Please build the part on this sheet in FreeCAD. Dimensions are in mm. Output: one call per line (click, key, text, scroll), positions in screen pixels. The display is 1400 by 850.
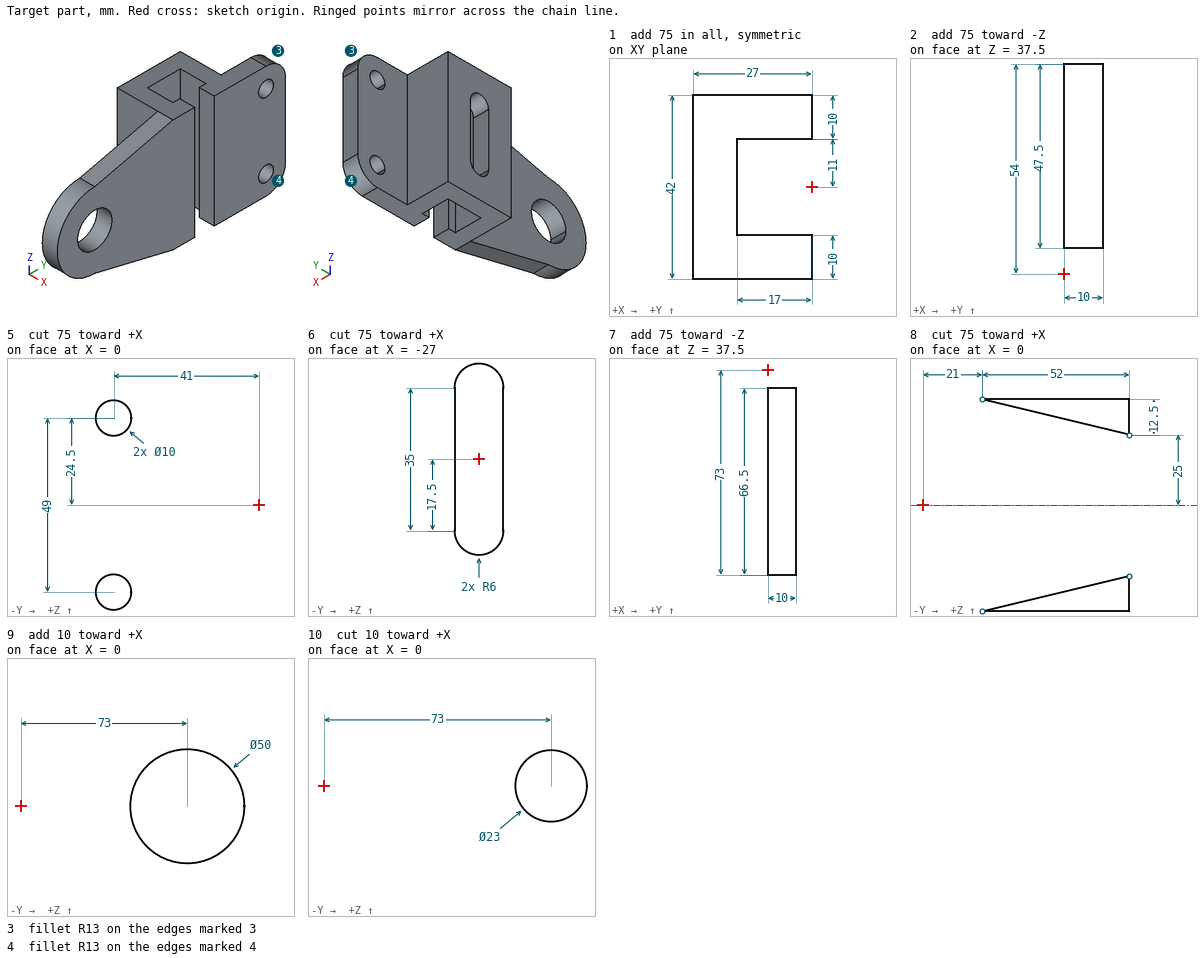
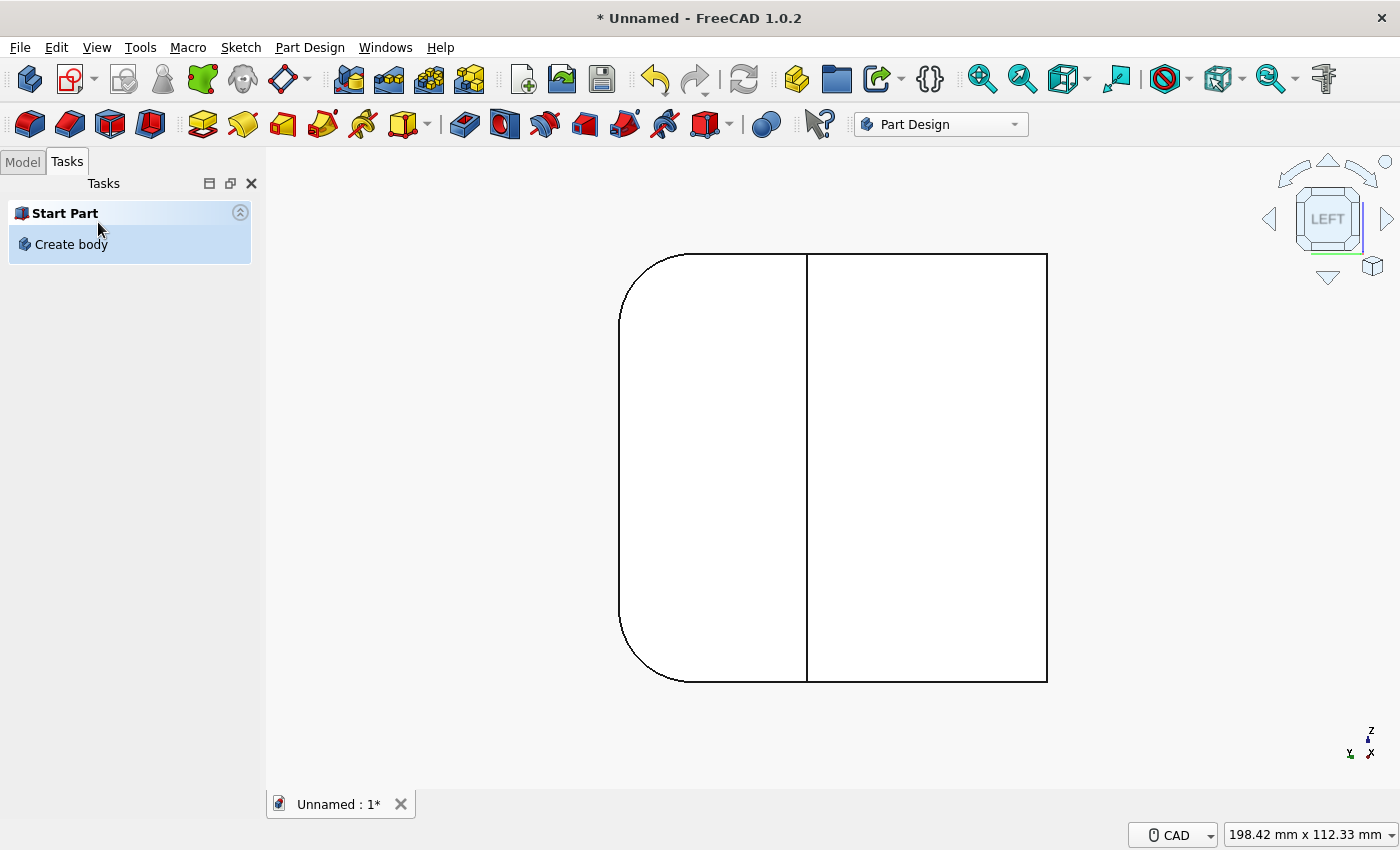
click(713, 406)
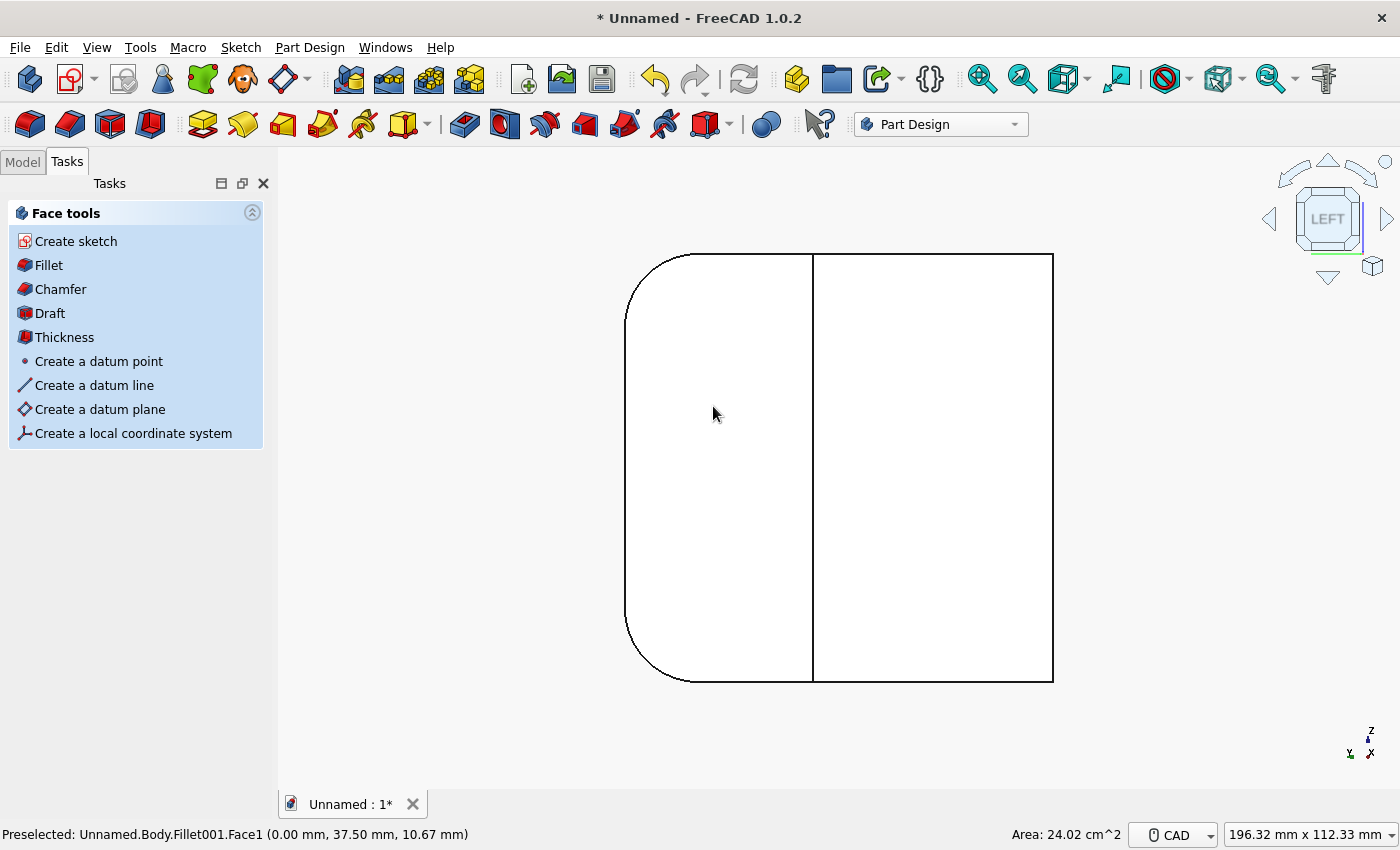
click(70, 80)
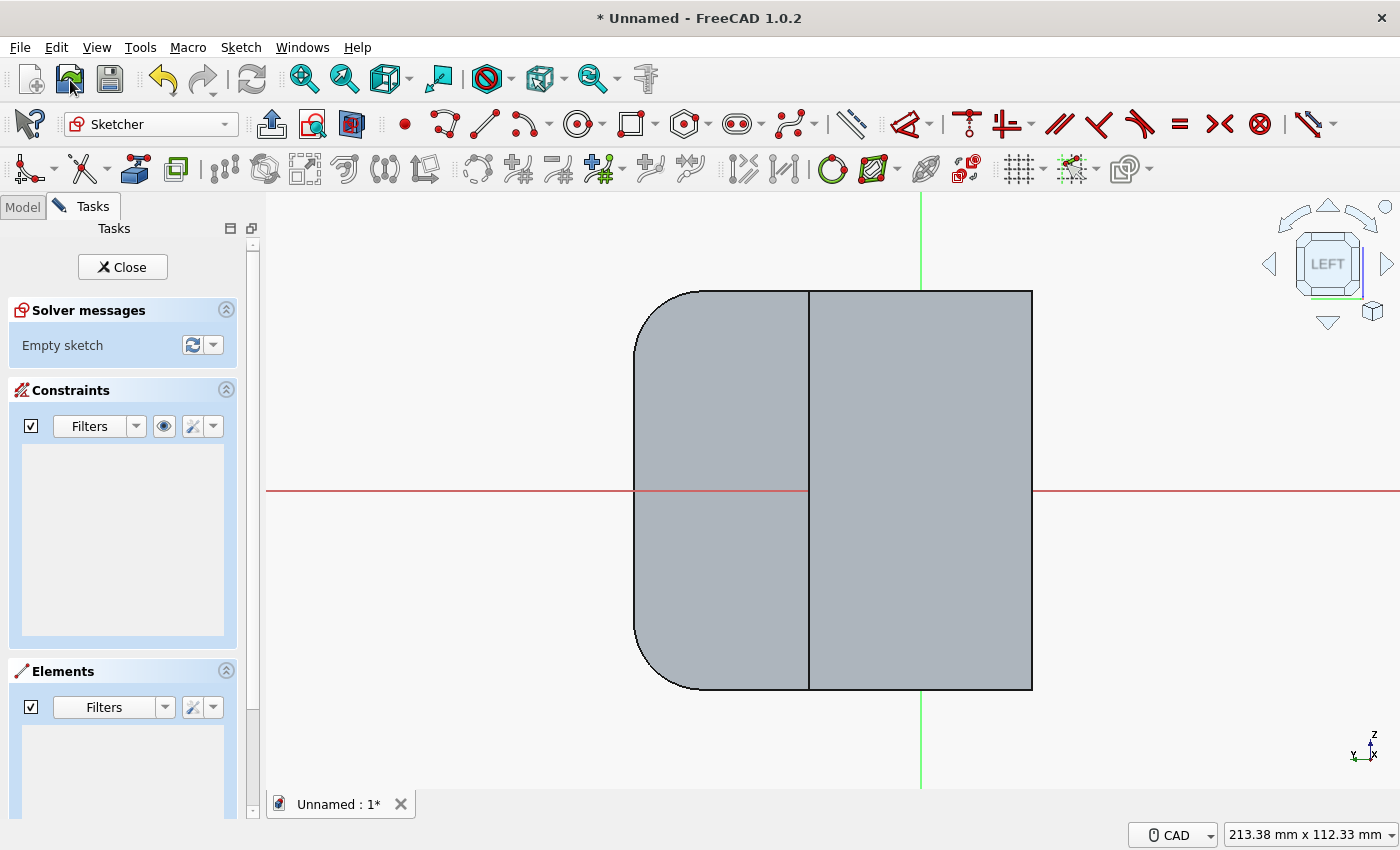
key(q)
key(s)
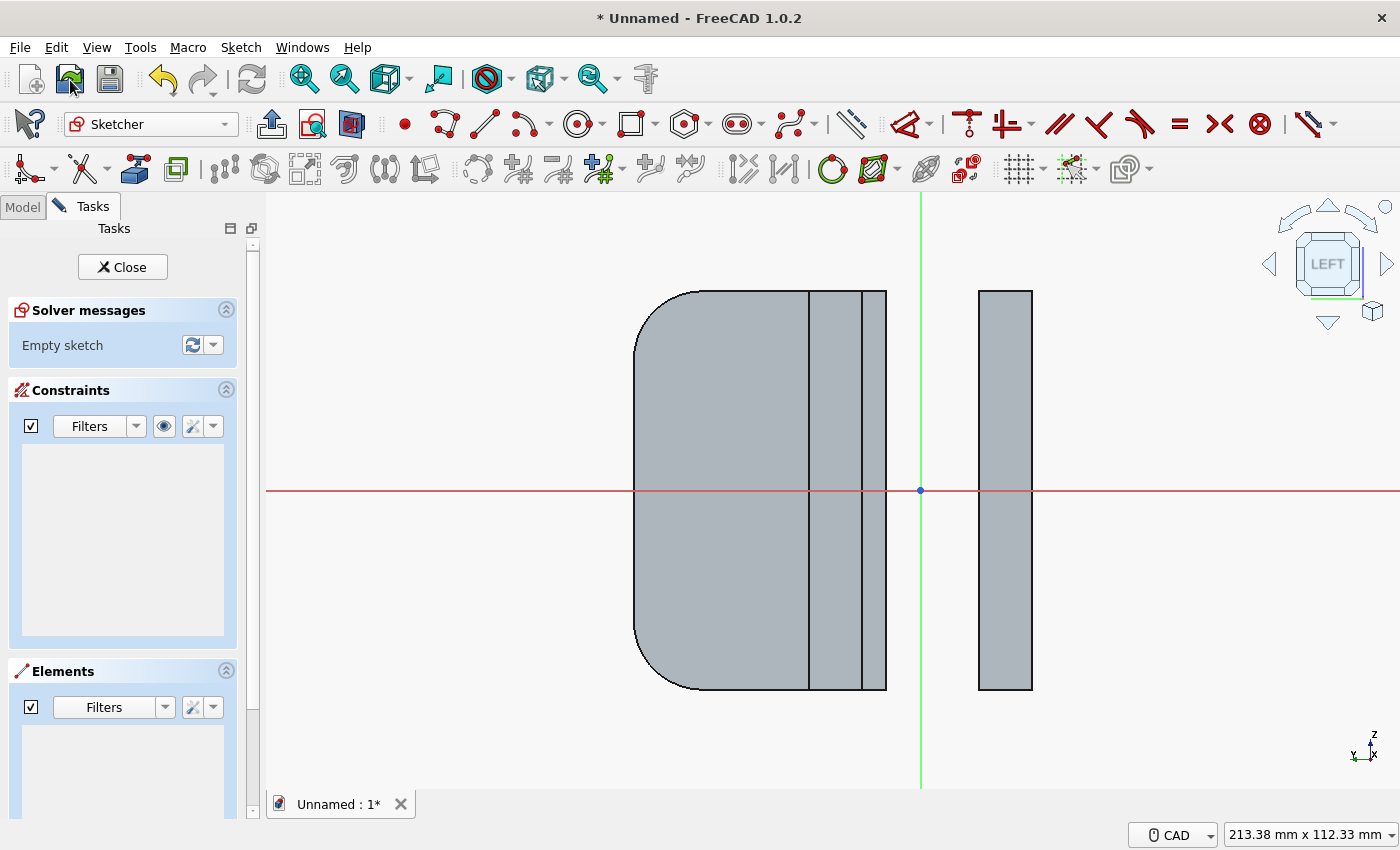
key(g)
key(c)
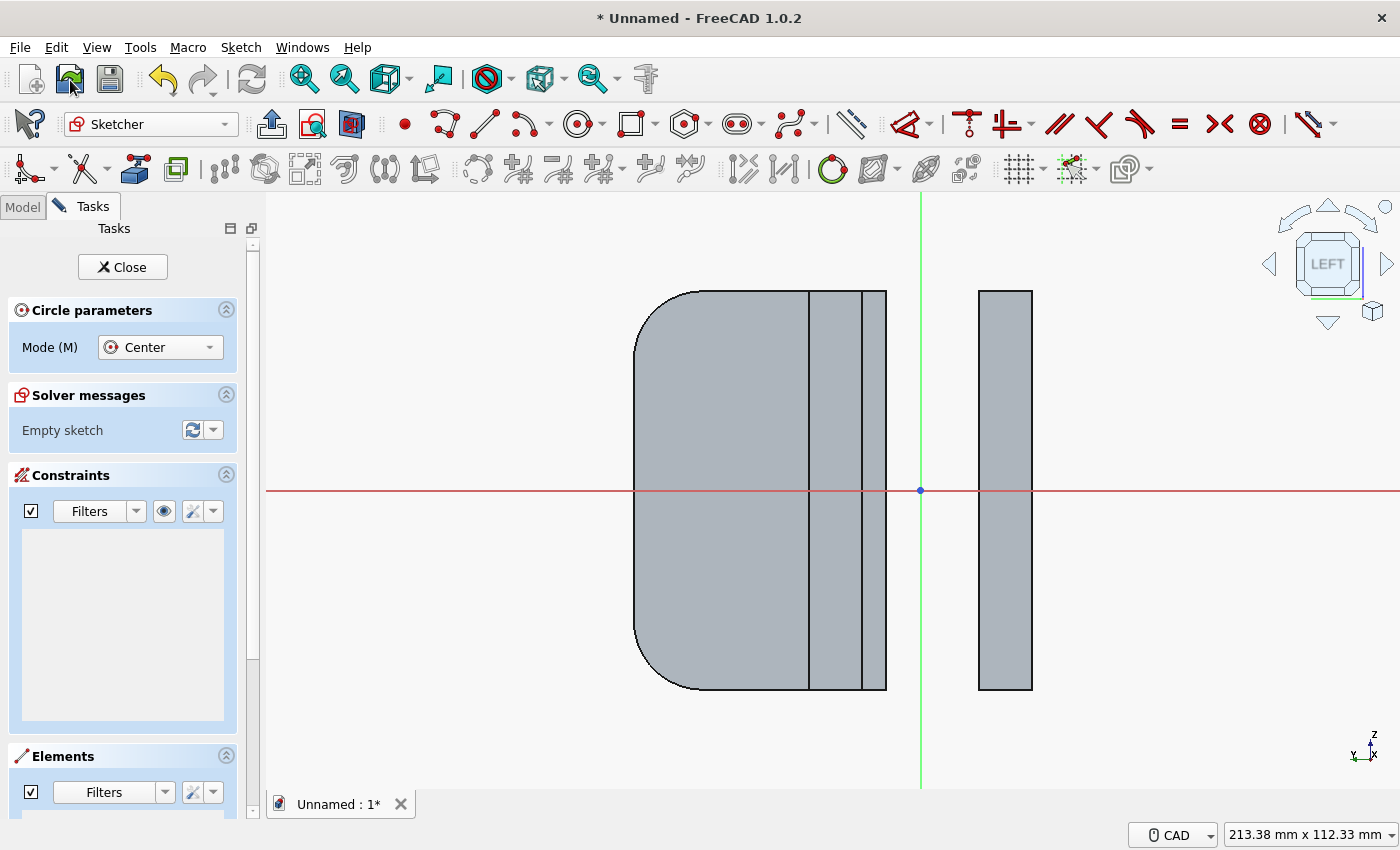
click(703, 360)
click(722, 342)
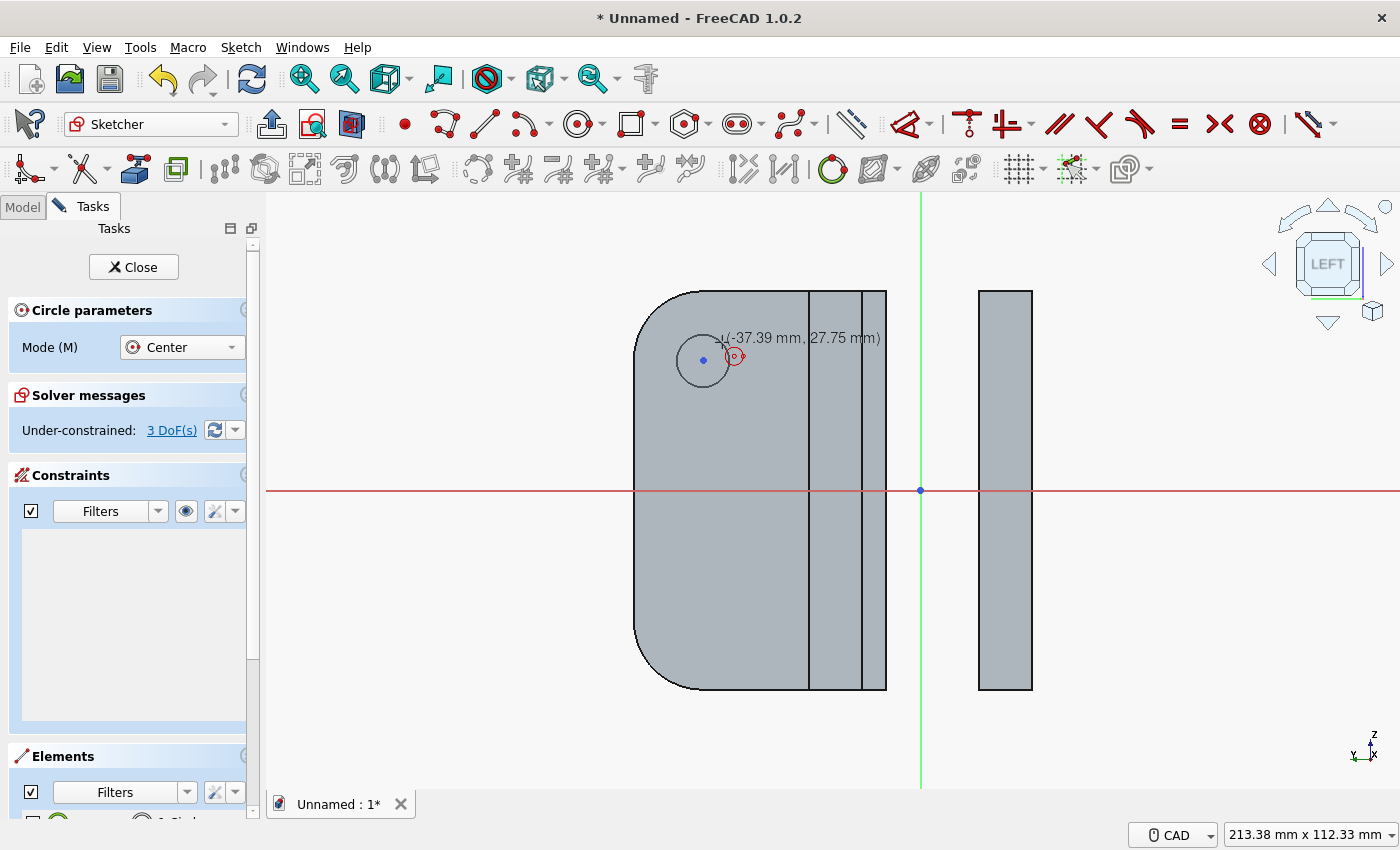
click(703, 621)
click(722, 602)
key(Escape)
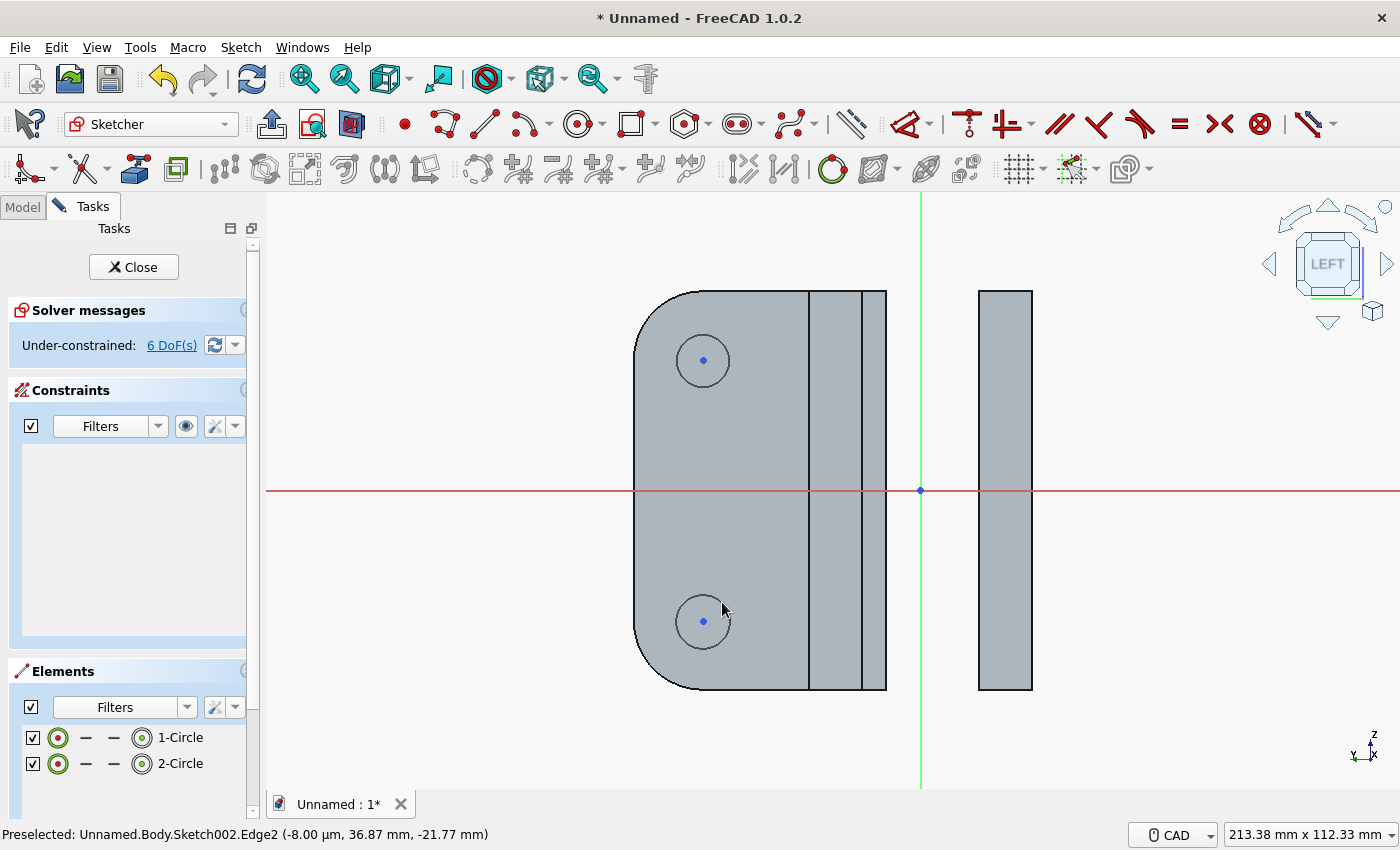
click(721, 342)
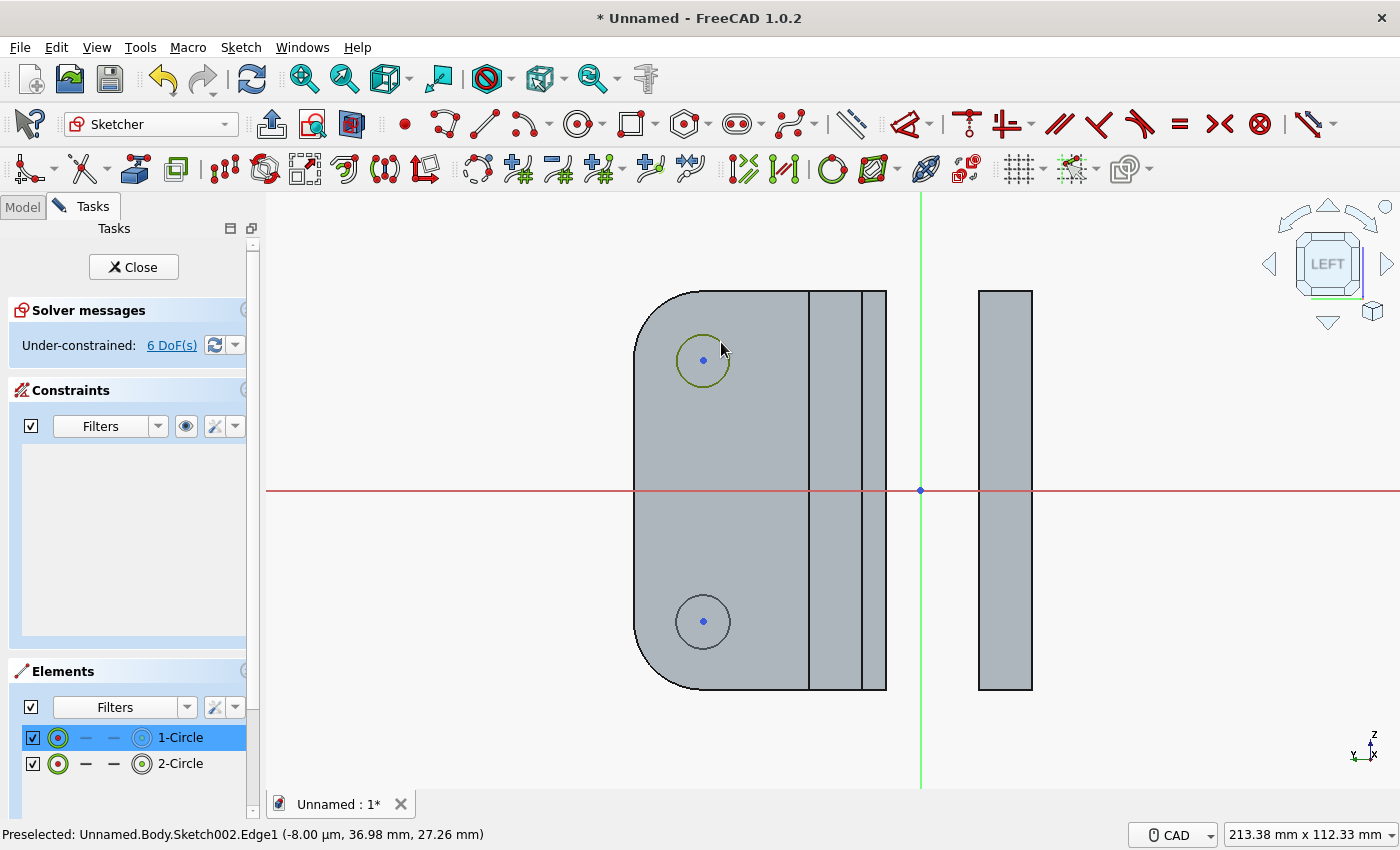
click(722, 603)